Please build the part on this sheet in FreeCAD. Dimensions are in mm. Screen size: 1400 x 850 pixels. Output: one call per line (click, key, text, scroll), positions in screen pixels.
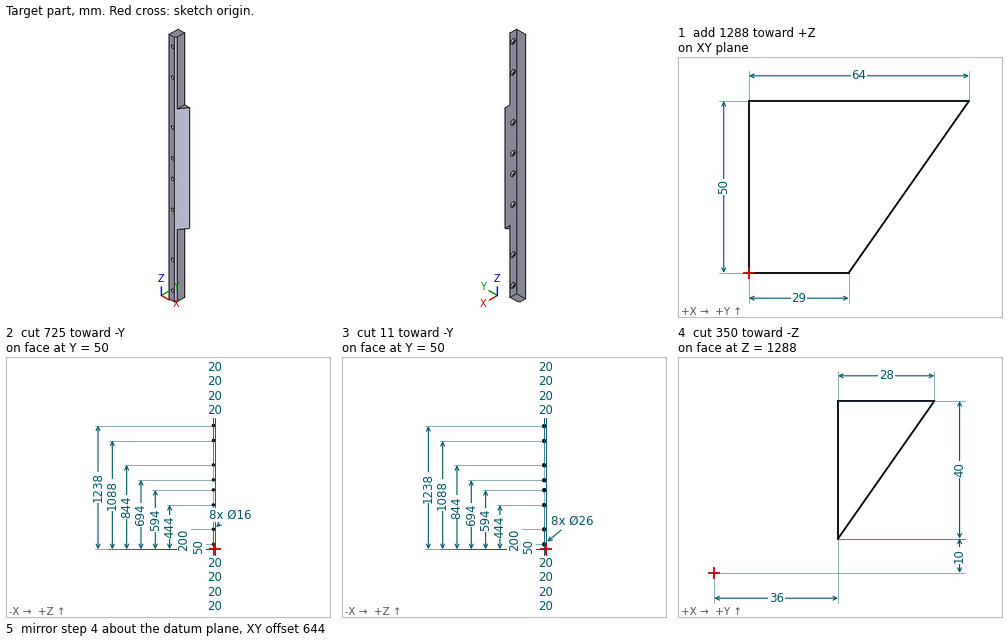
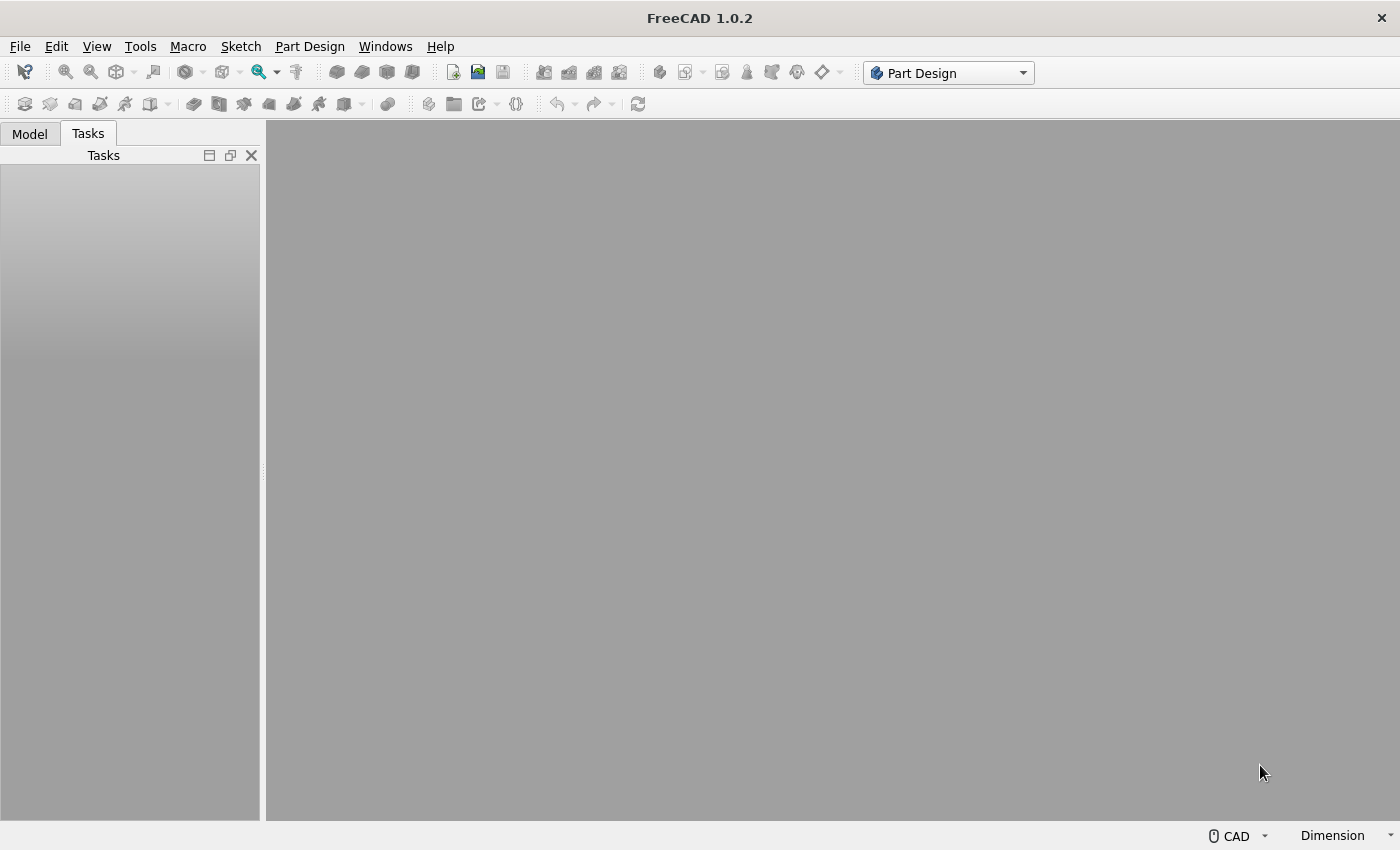
click(453, 72)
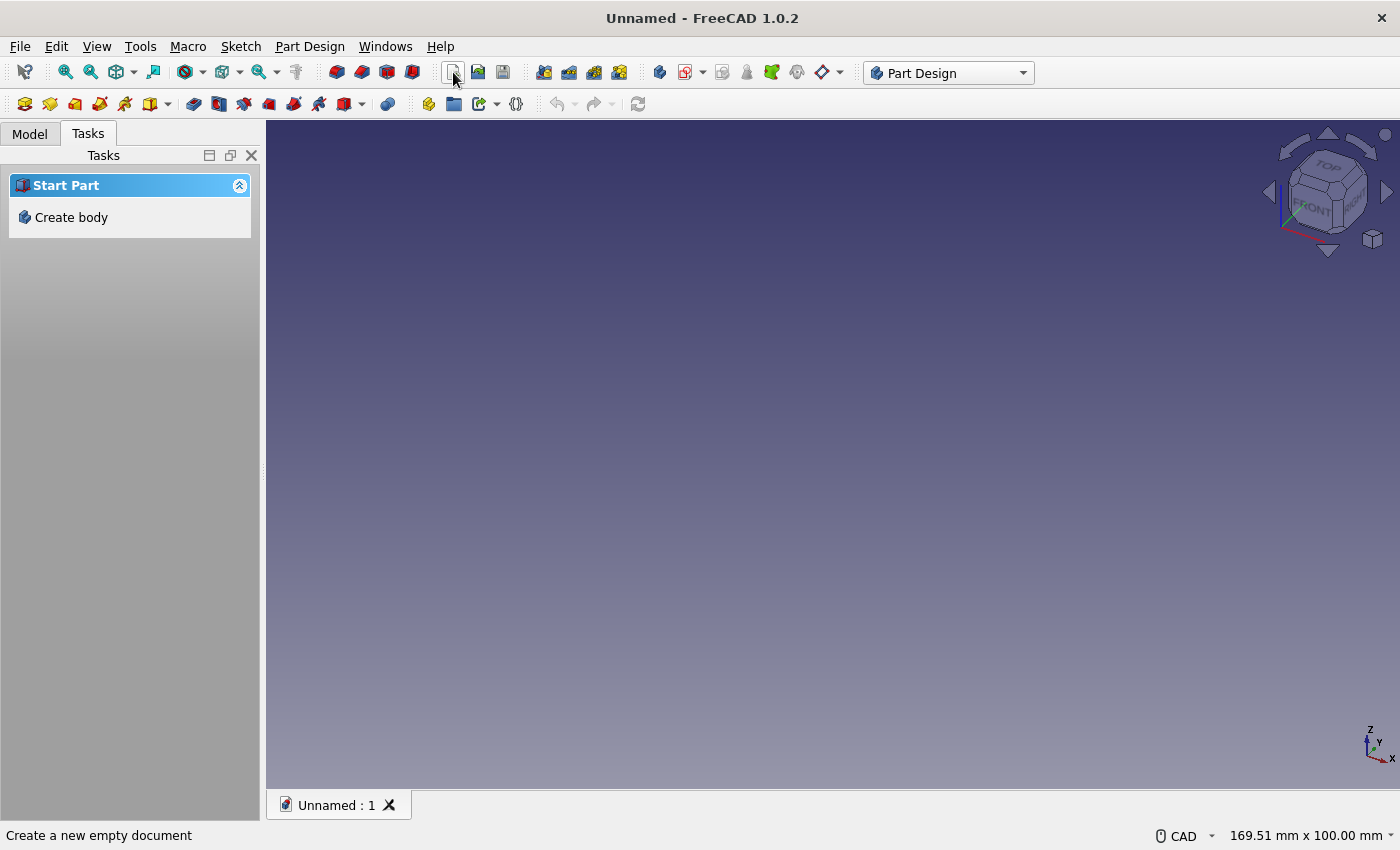
click(684, 72)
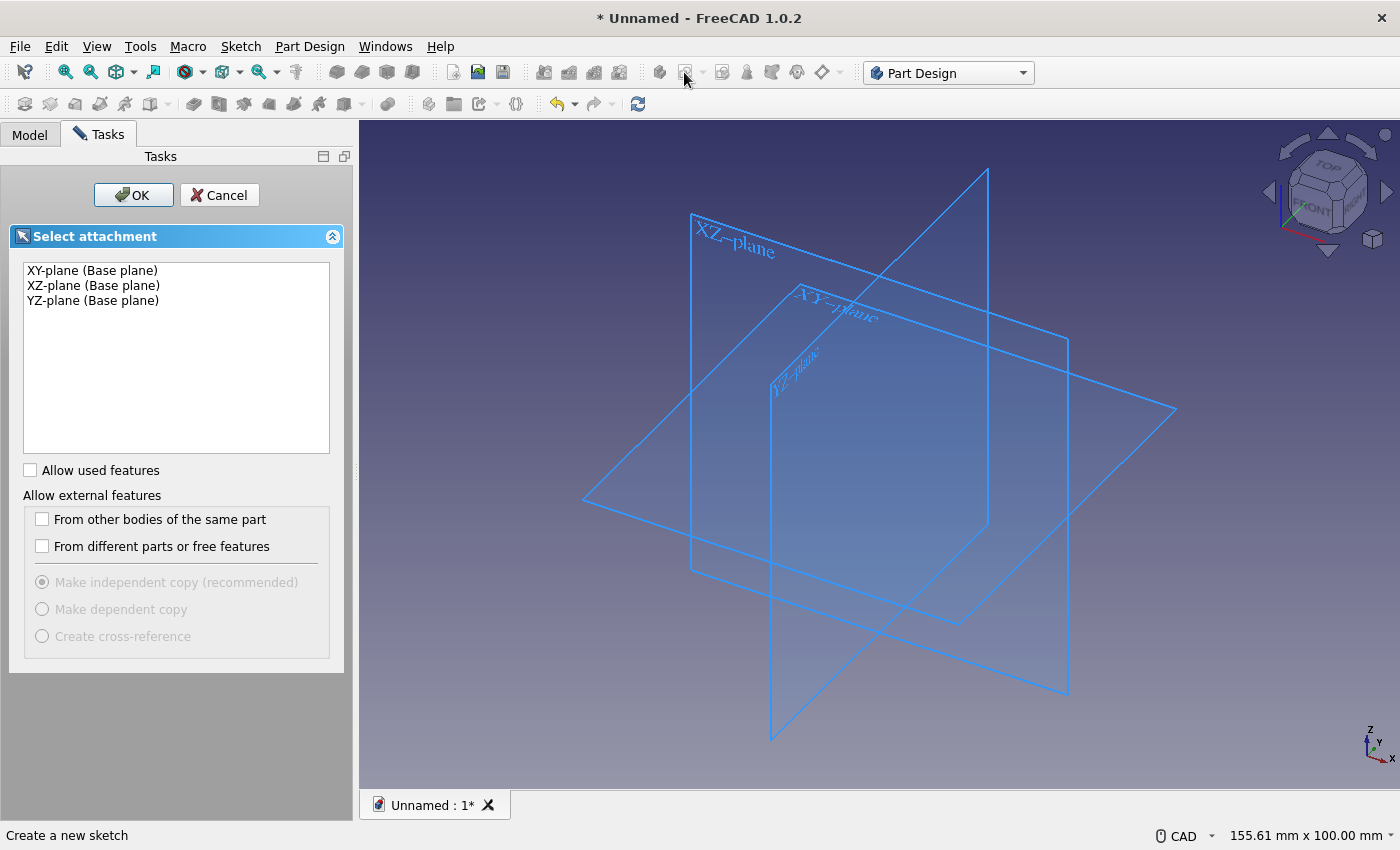
click(84, 270)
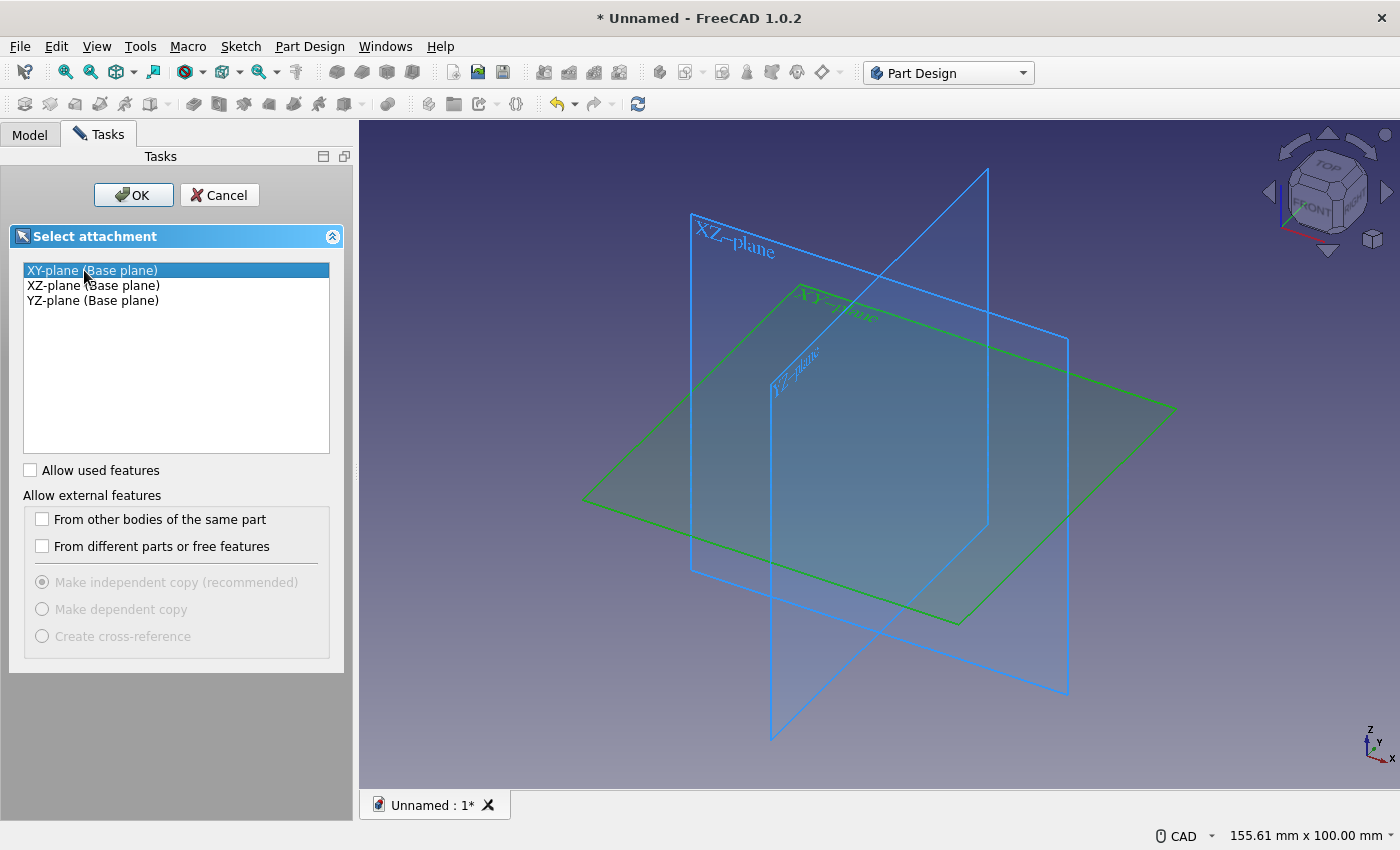
click(134, 195)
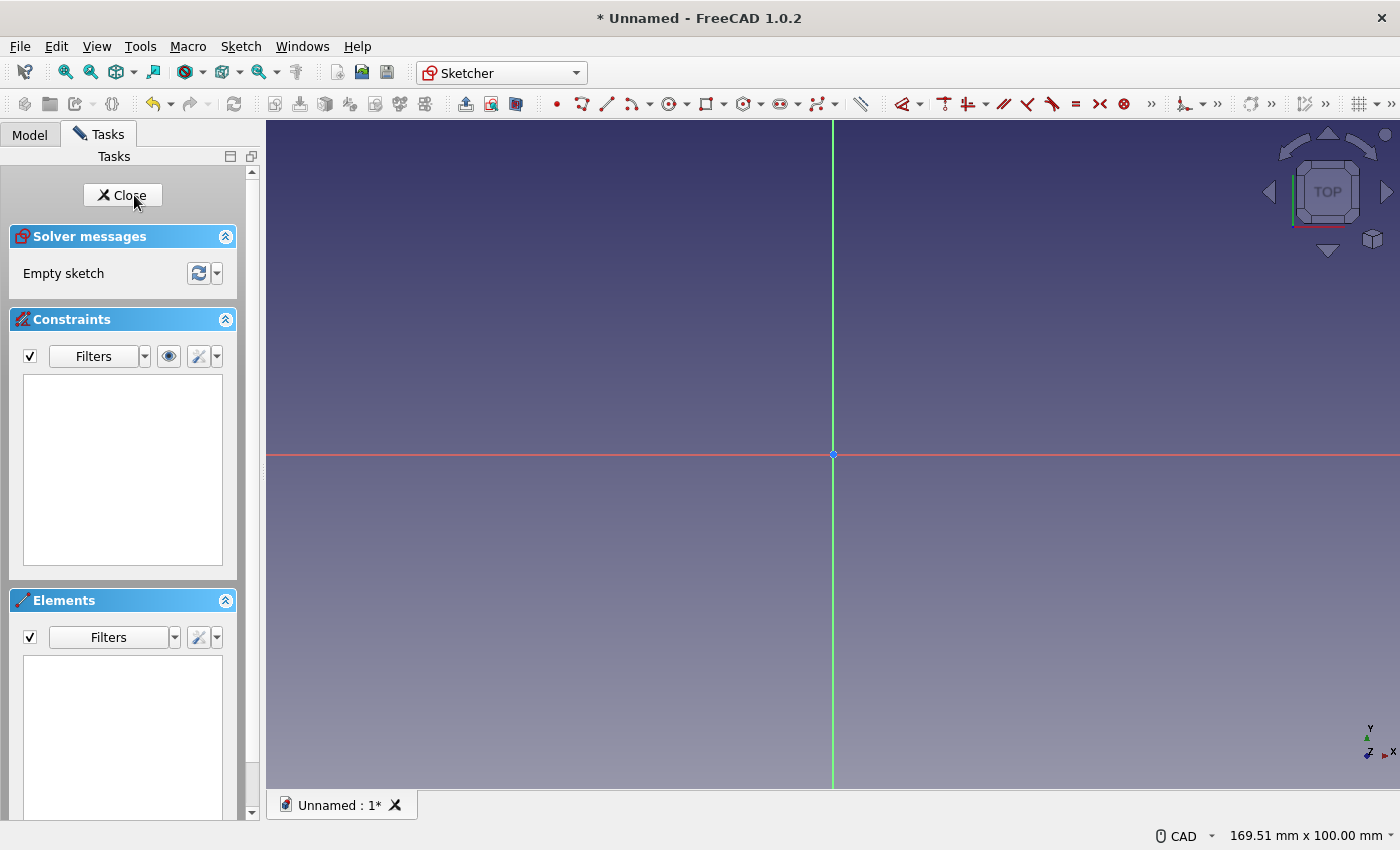
scroll(294, 761, down, 1)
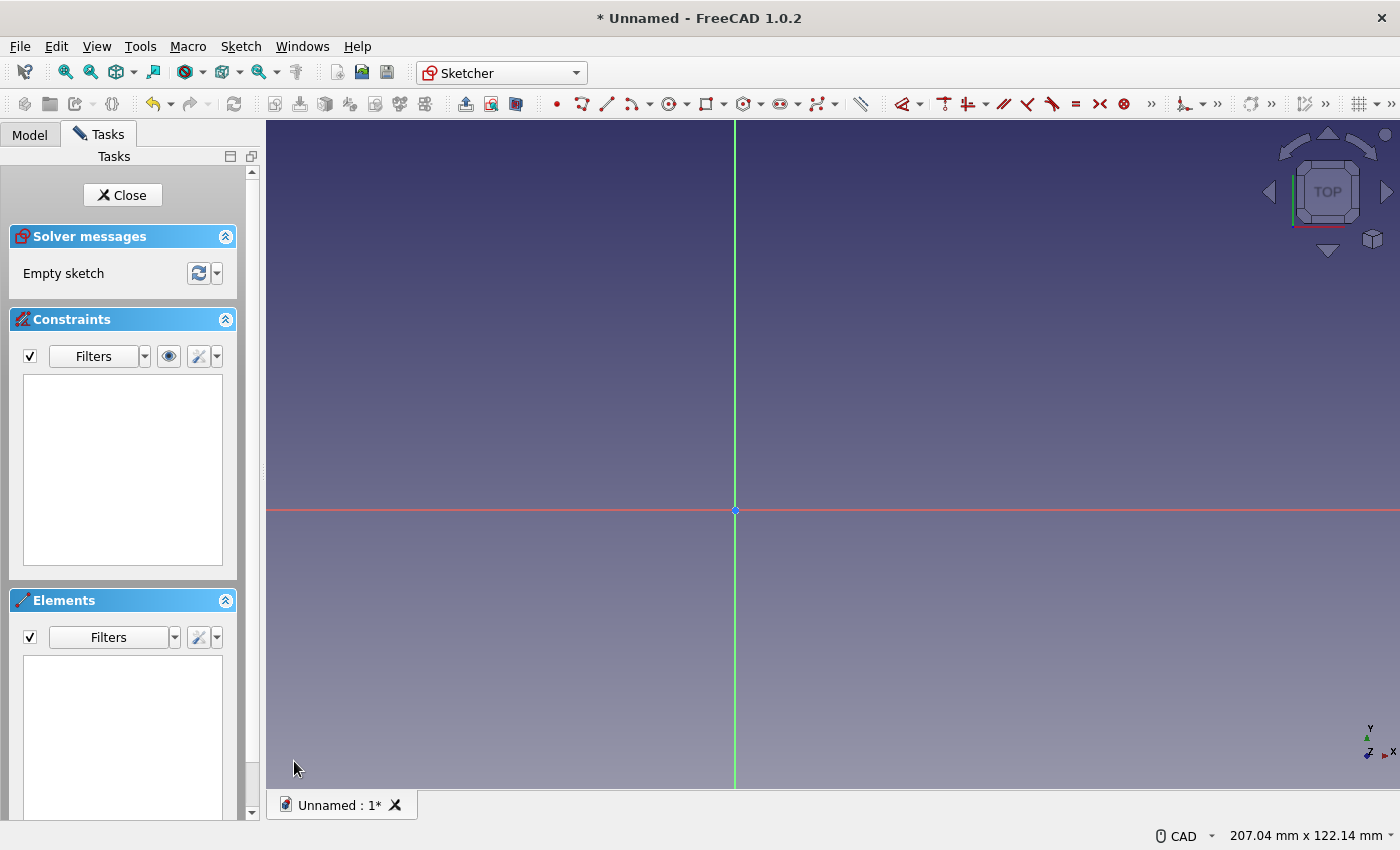
scroll(1208, 208, up, 2)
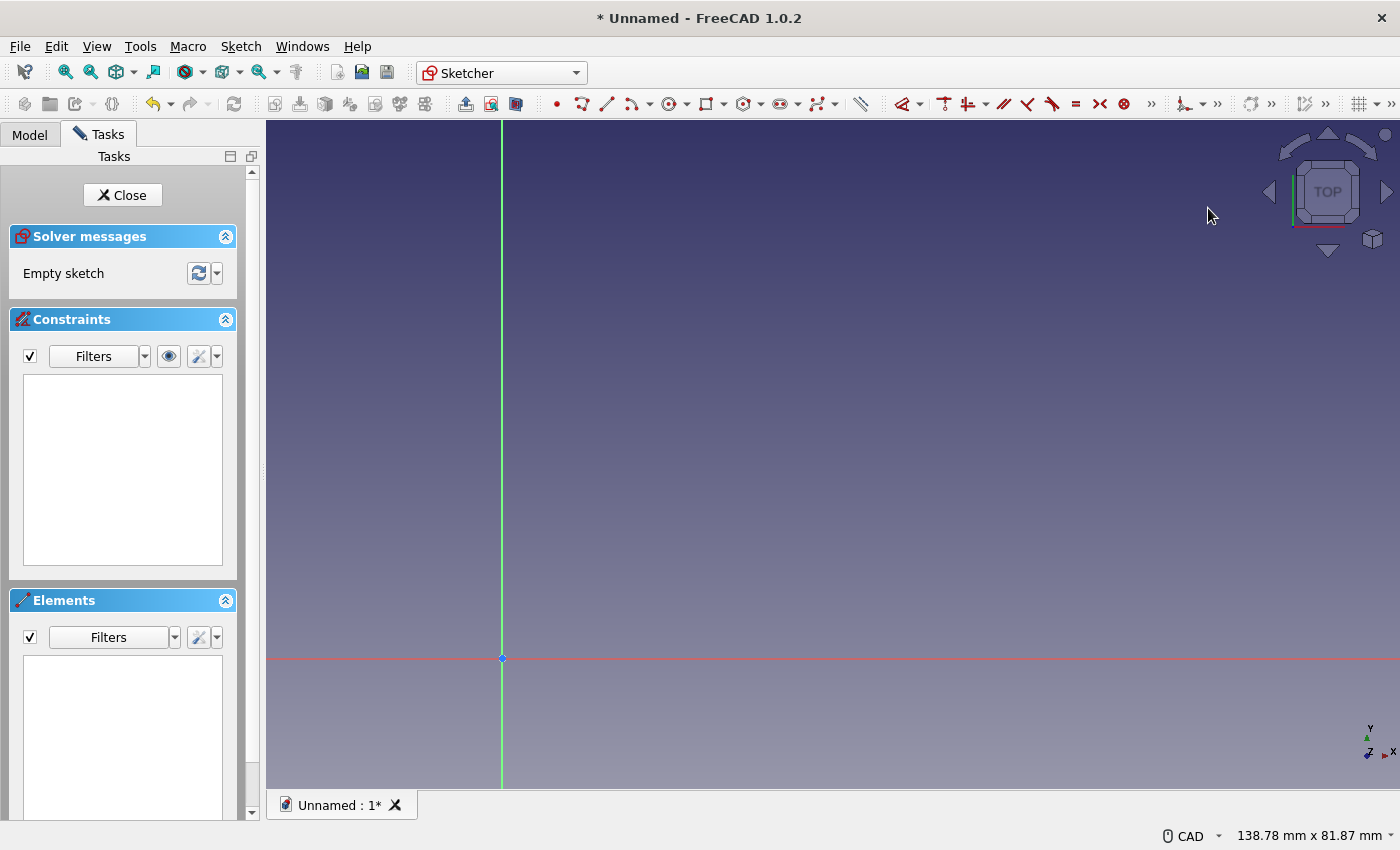
click(582, 104)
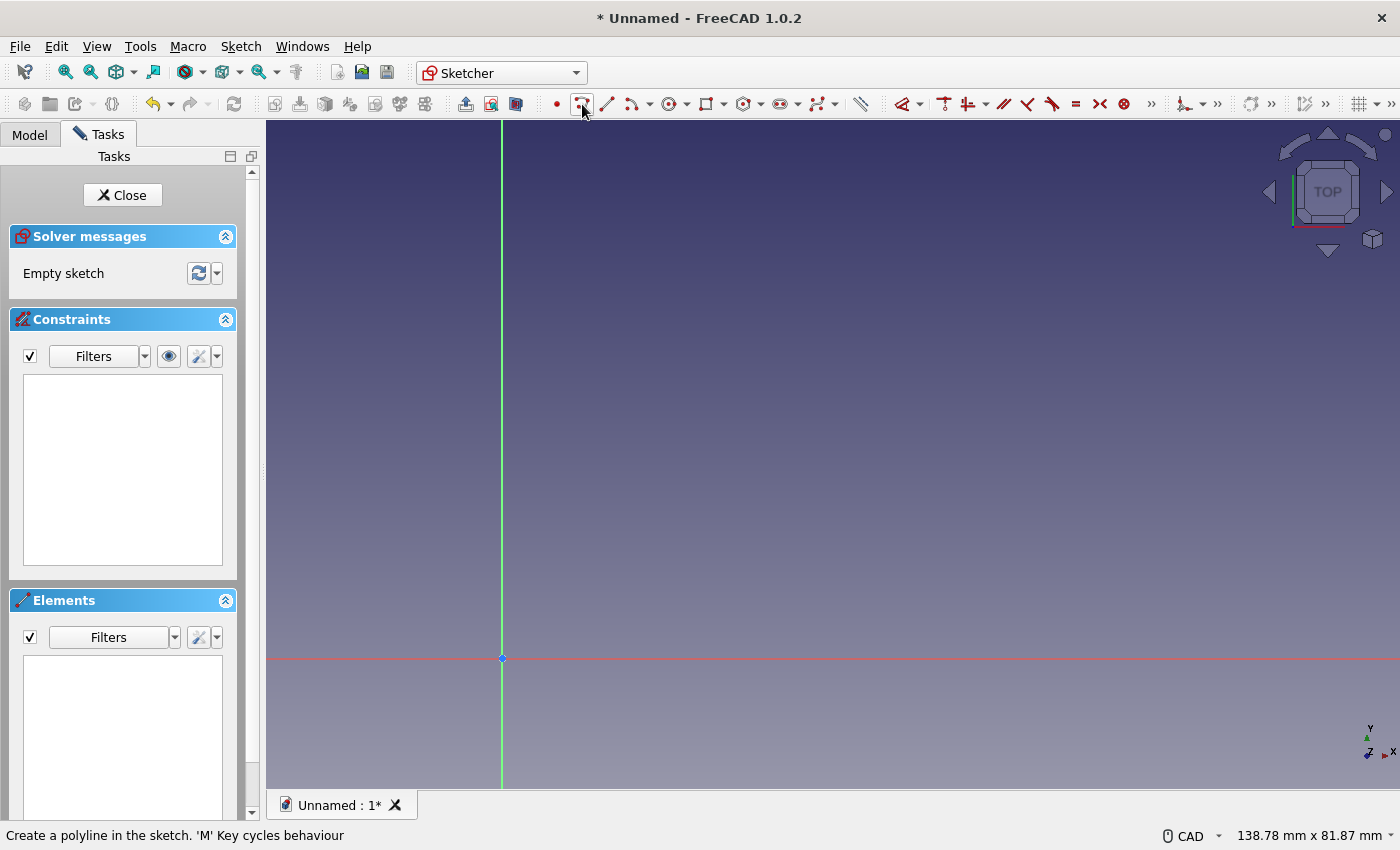
click(502, 659)
click(739, 650)
click(1025, 250)
click(511, 250)
click(502, 659)
key(Escape)
key(Escape)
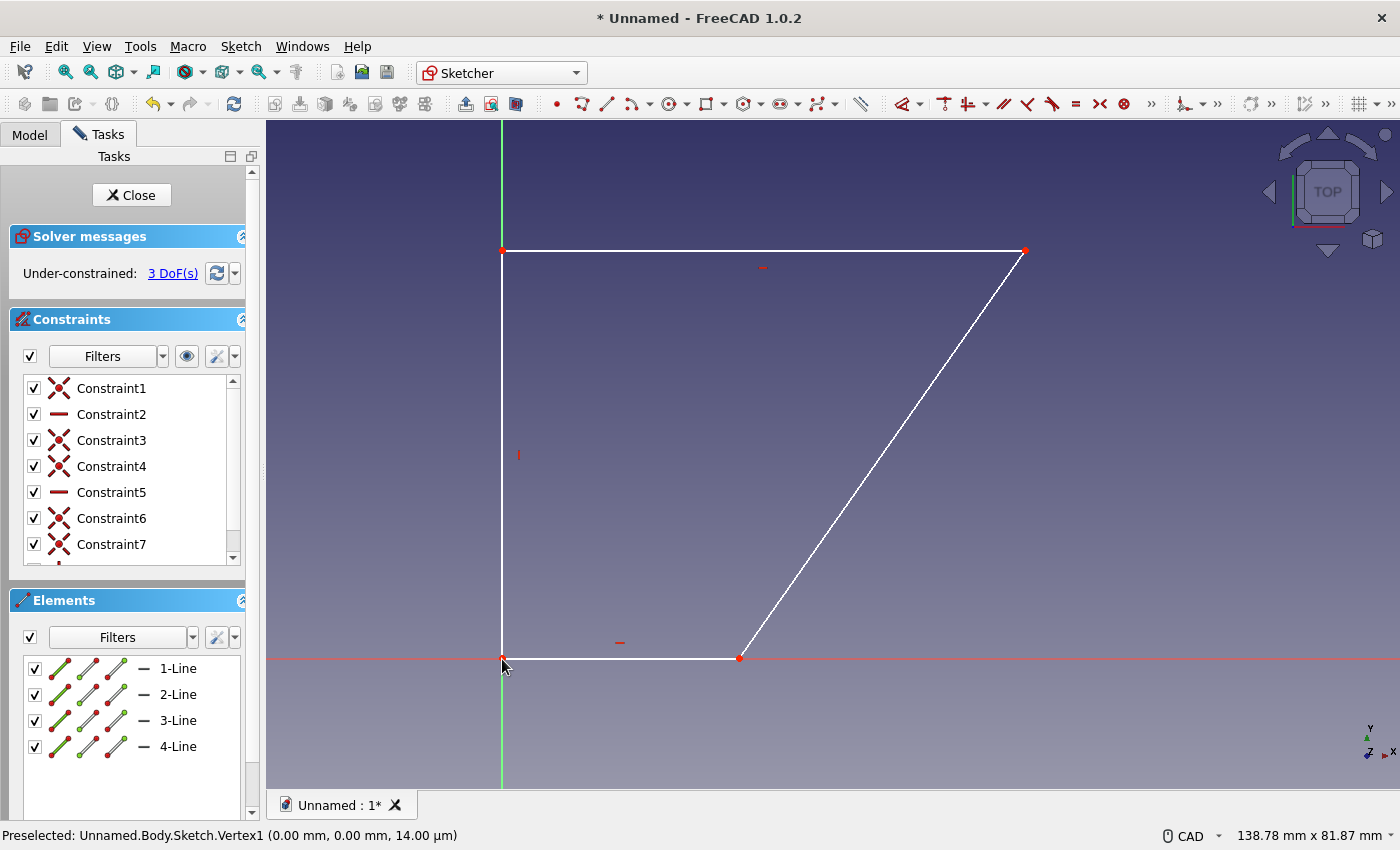
click(573, 659)